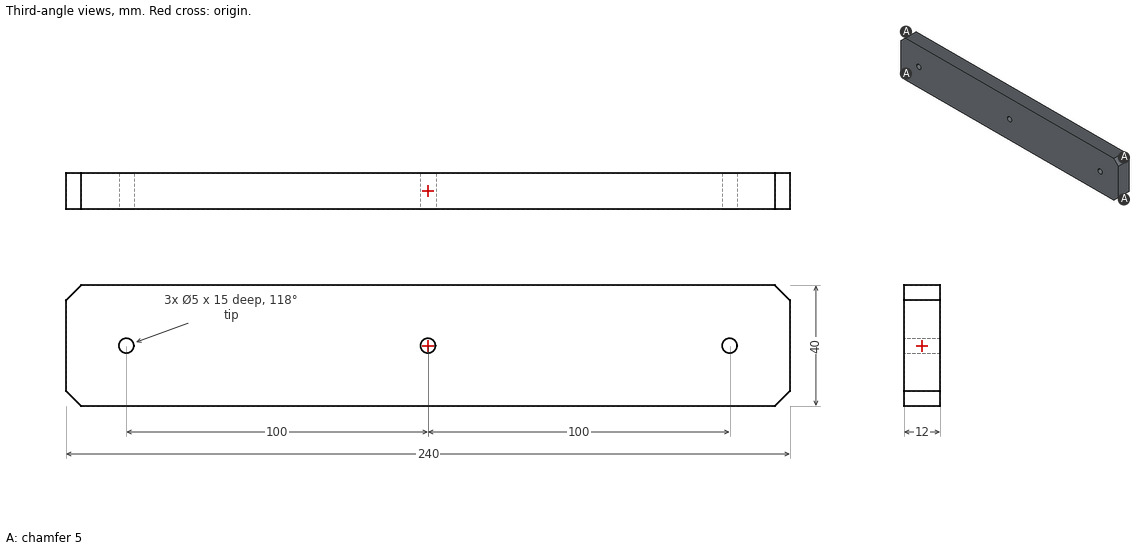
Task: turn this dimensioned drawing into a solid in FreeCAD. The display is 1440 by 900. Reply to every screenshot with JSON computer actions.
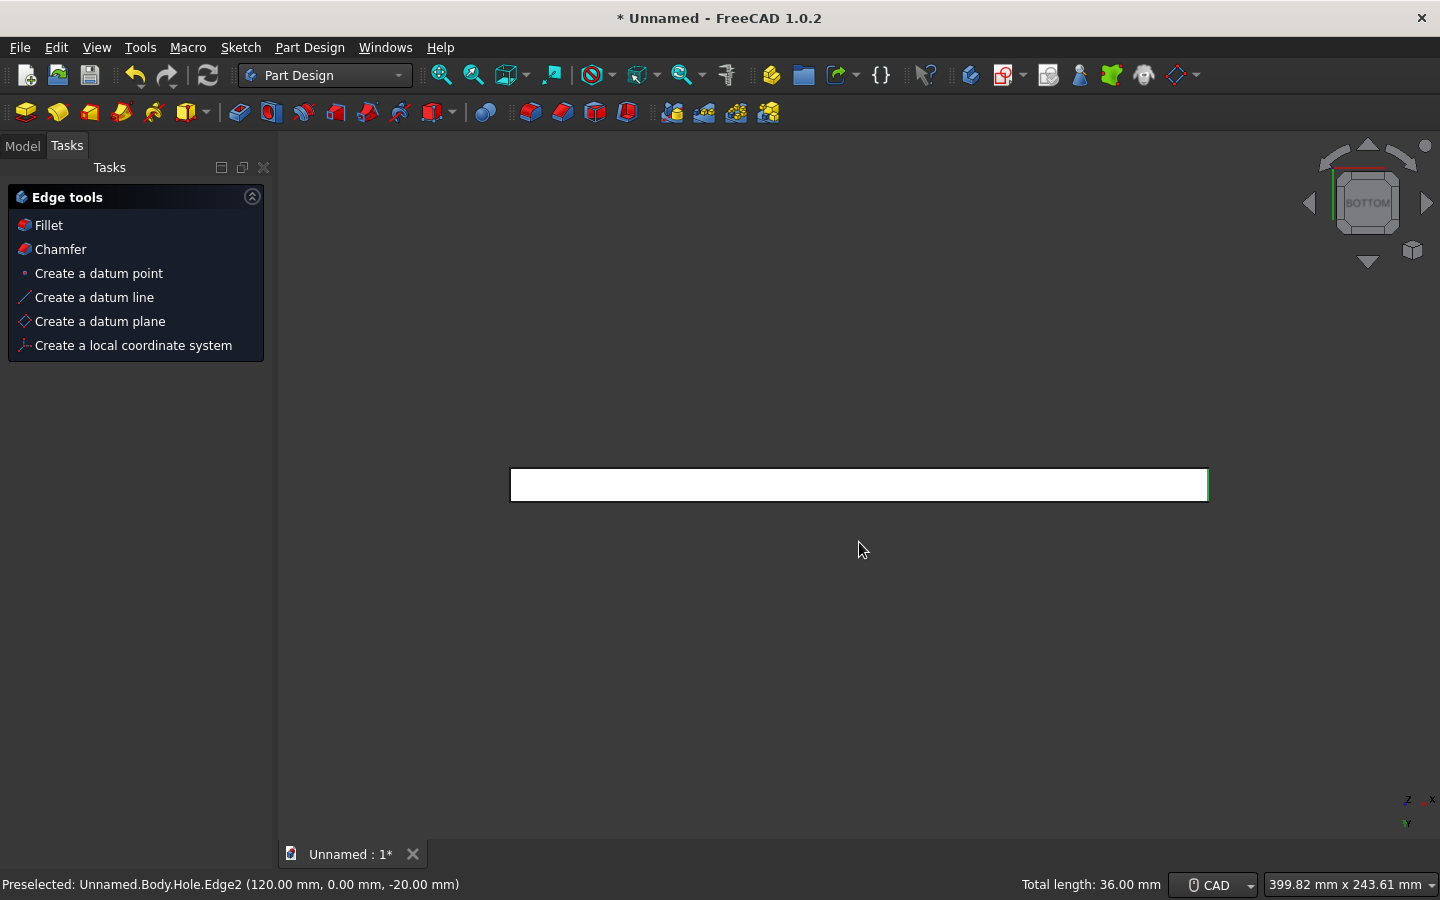
{"action": "left_click", "coordinate": [510, 484], "text": "ctrl"}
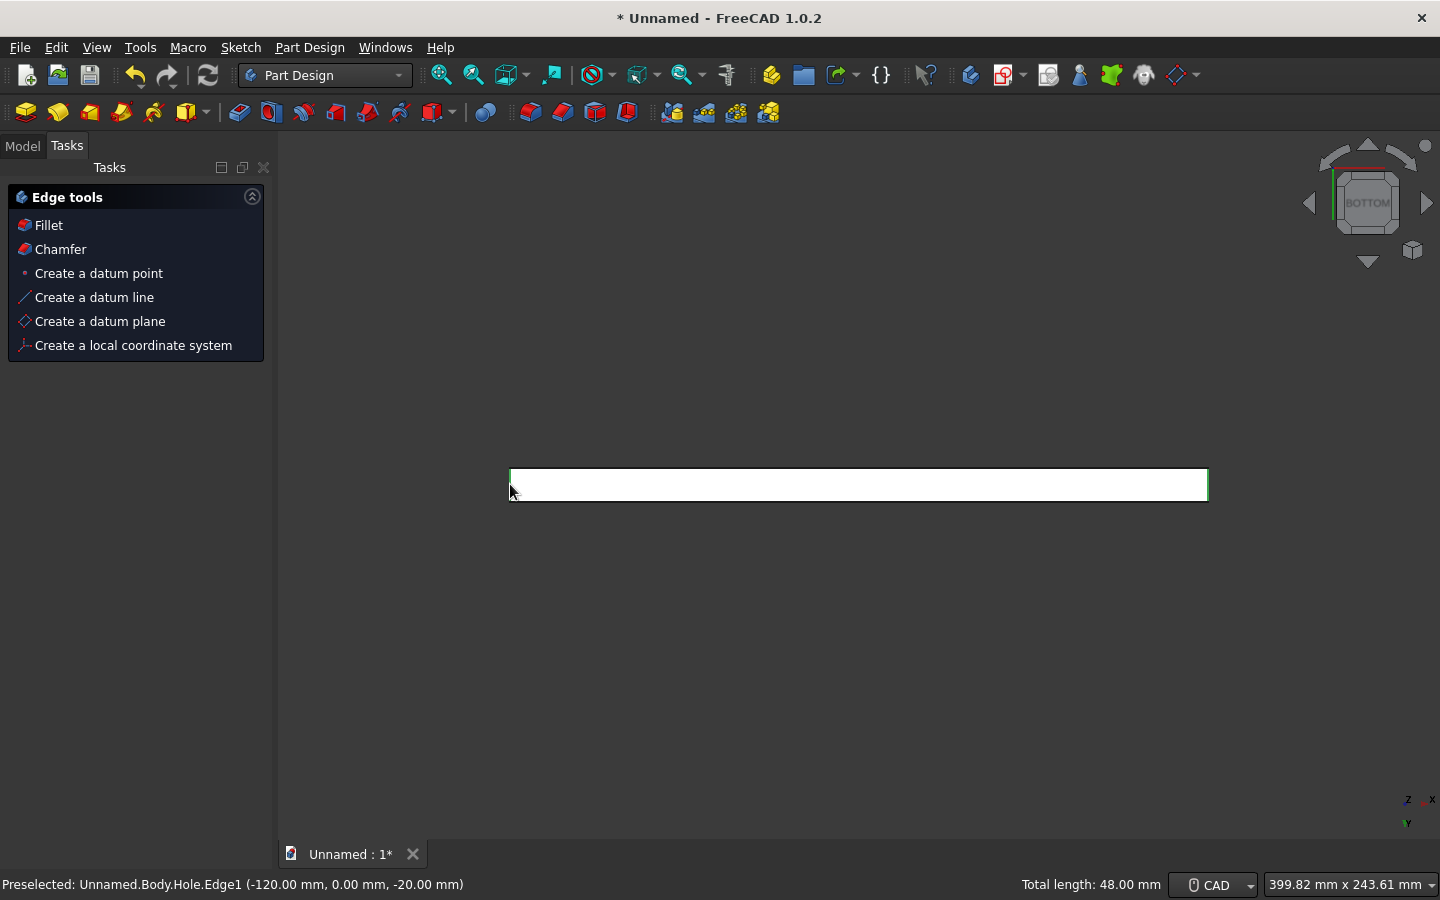
{"action": "left_click", "coordinate": [564, 112]}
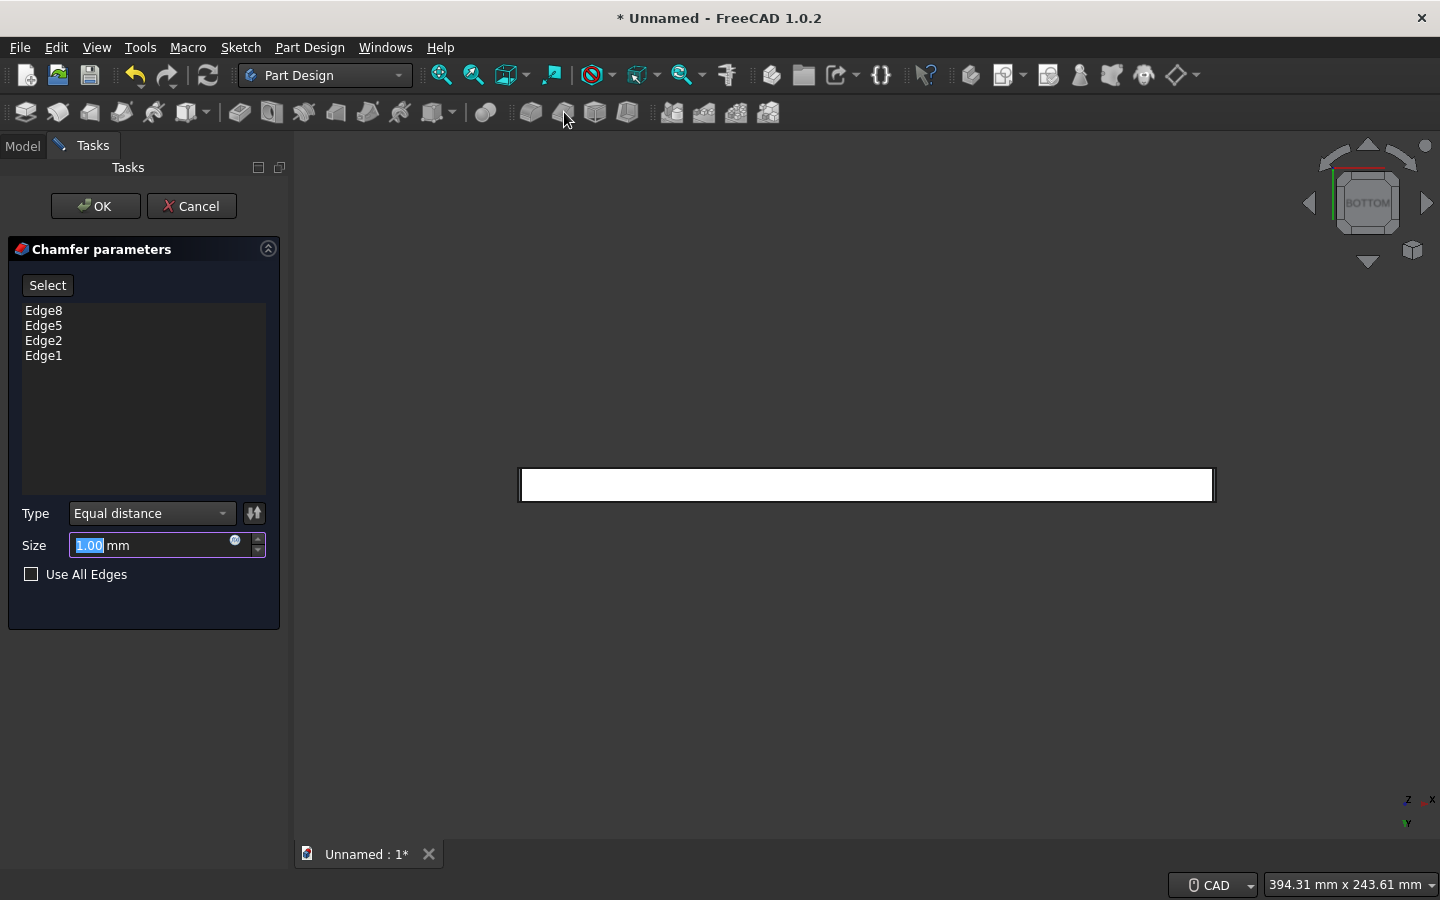
{"action": "type", "text": "5"}
{"action": "key", "text": "Tab"}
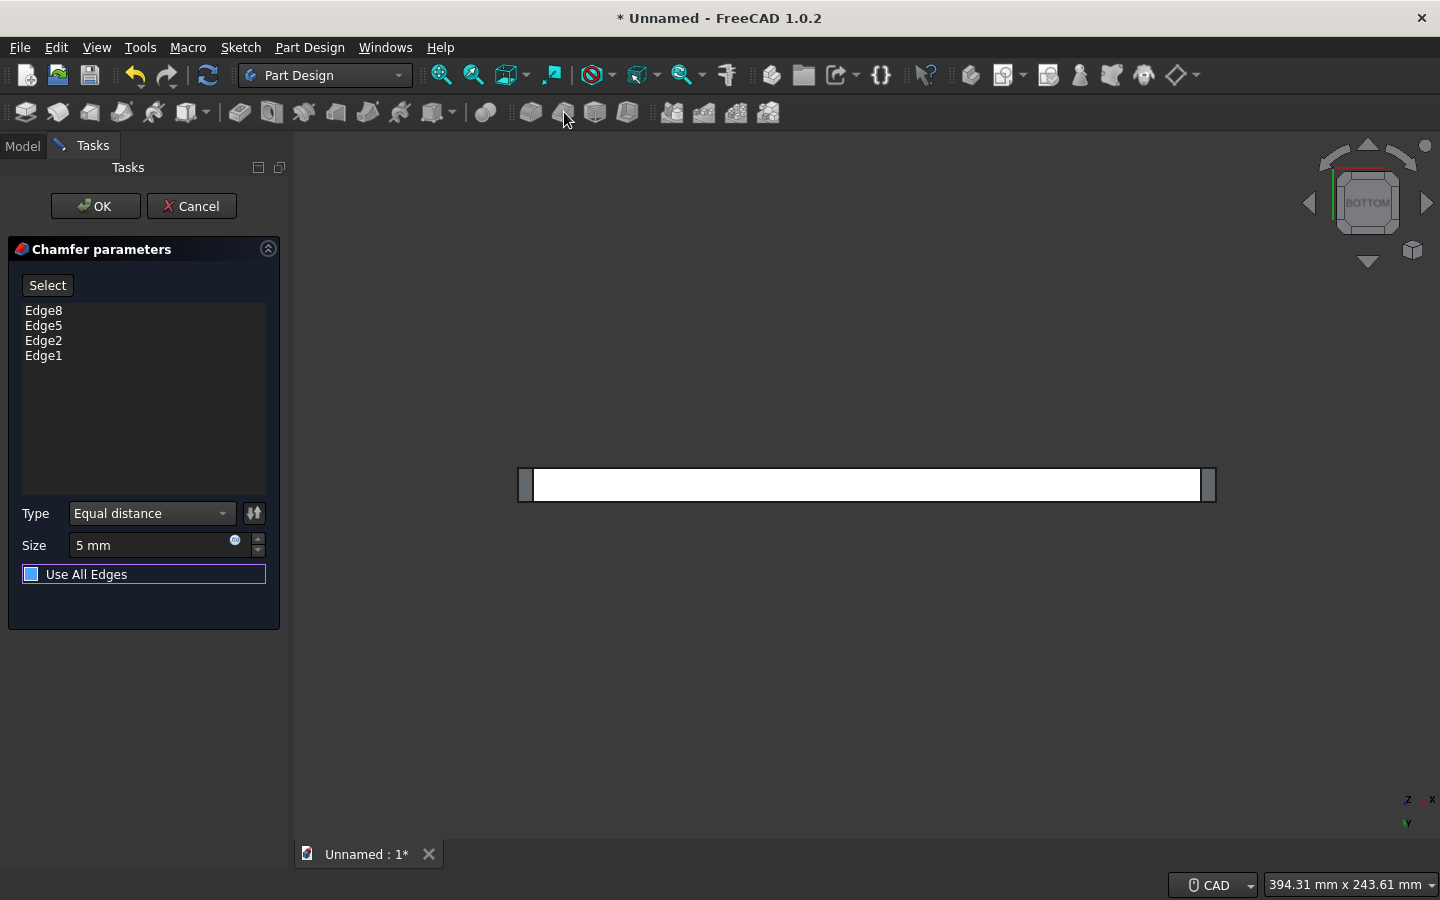
{"action": "left_click", "coordinate": [96, 206]}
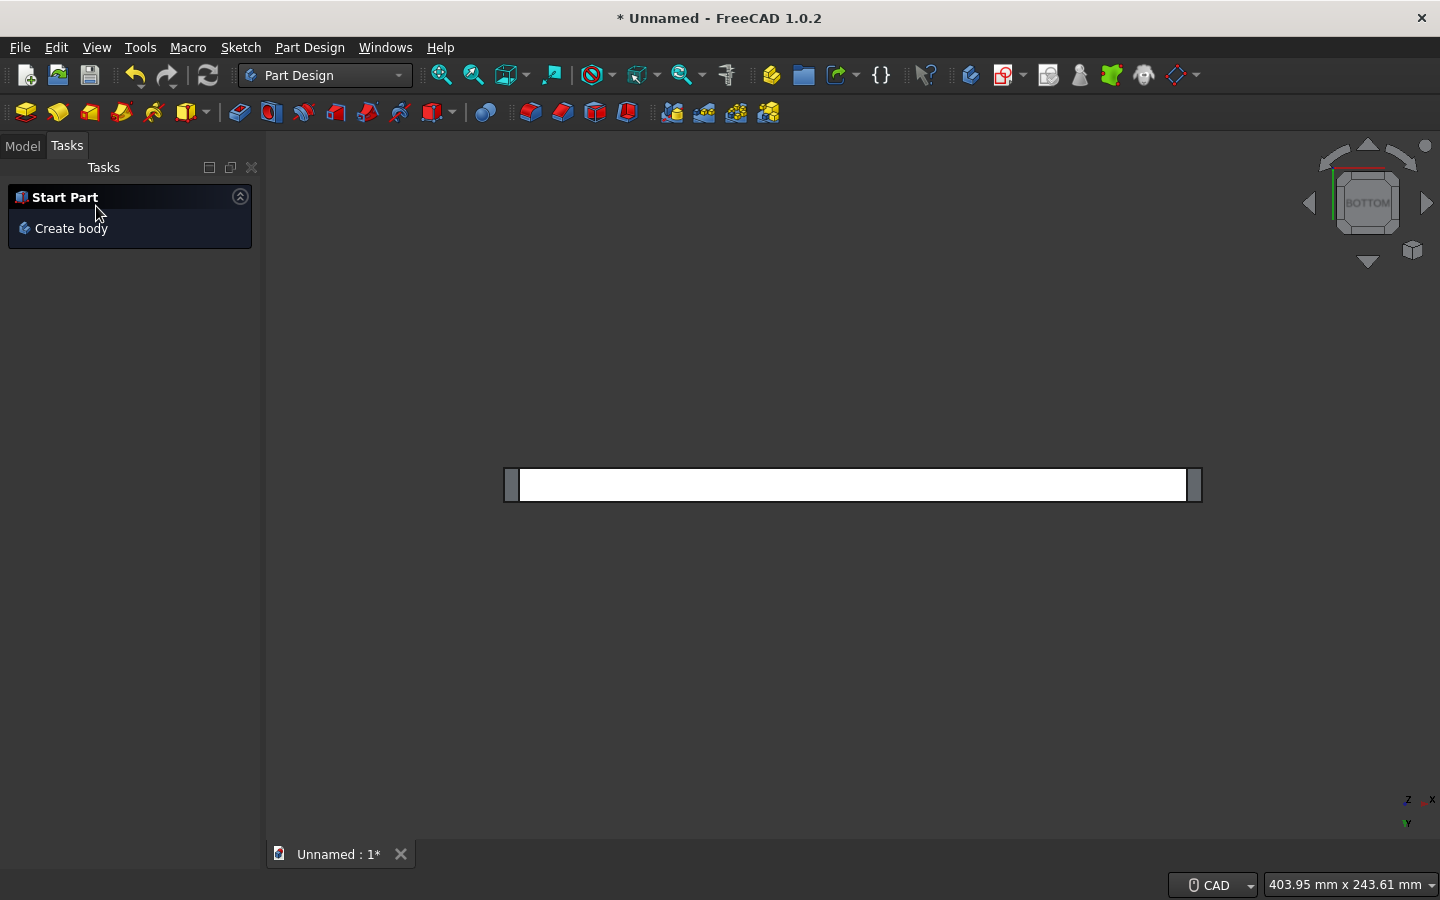
{"action": "key", "text": "0"}